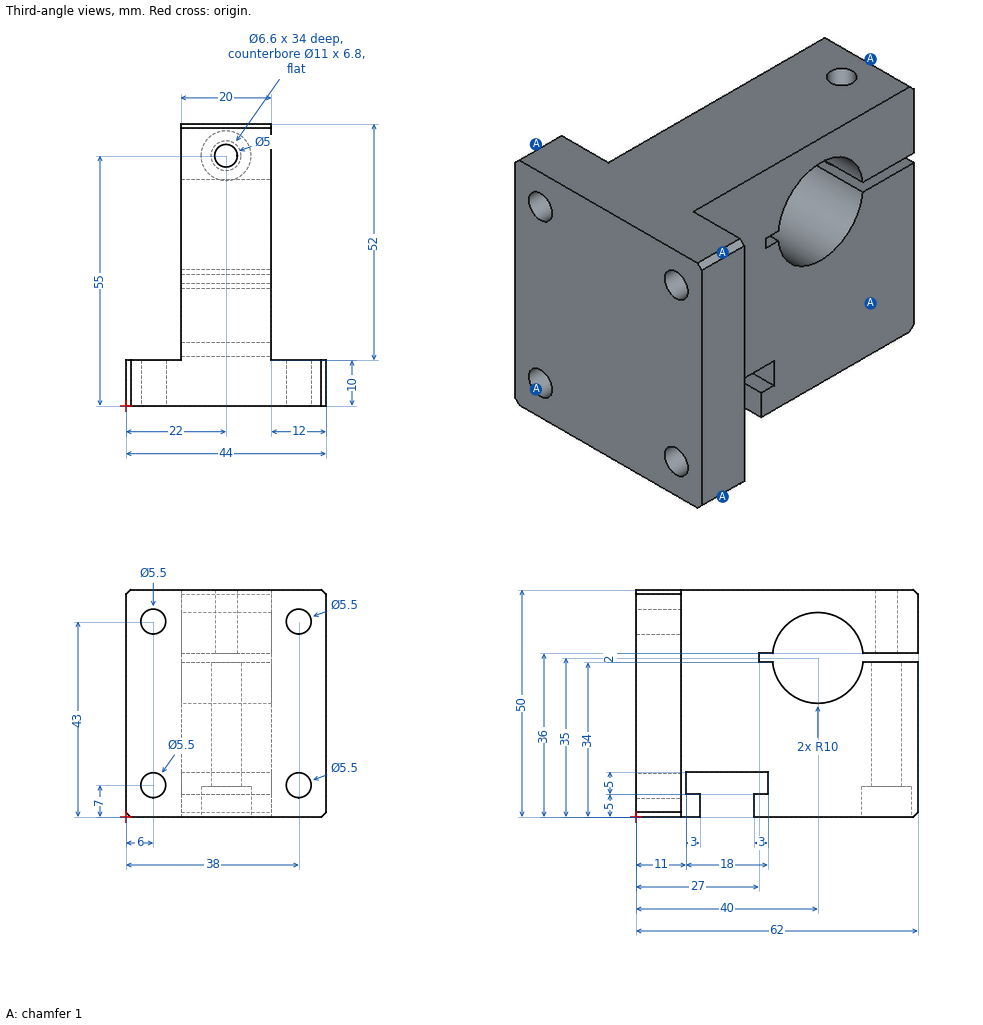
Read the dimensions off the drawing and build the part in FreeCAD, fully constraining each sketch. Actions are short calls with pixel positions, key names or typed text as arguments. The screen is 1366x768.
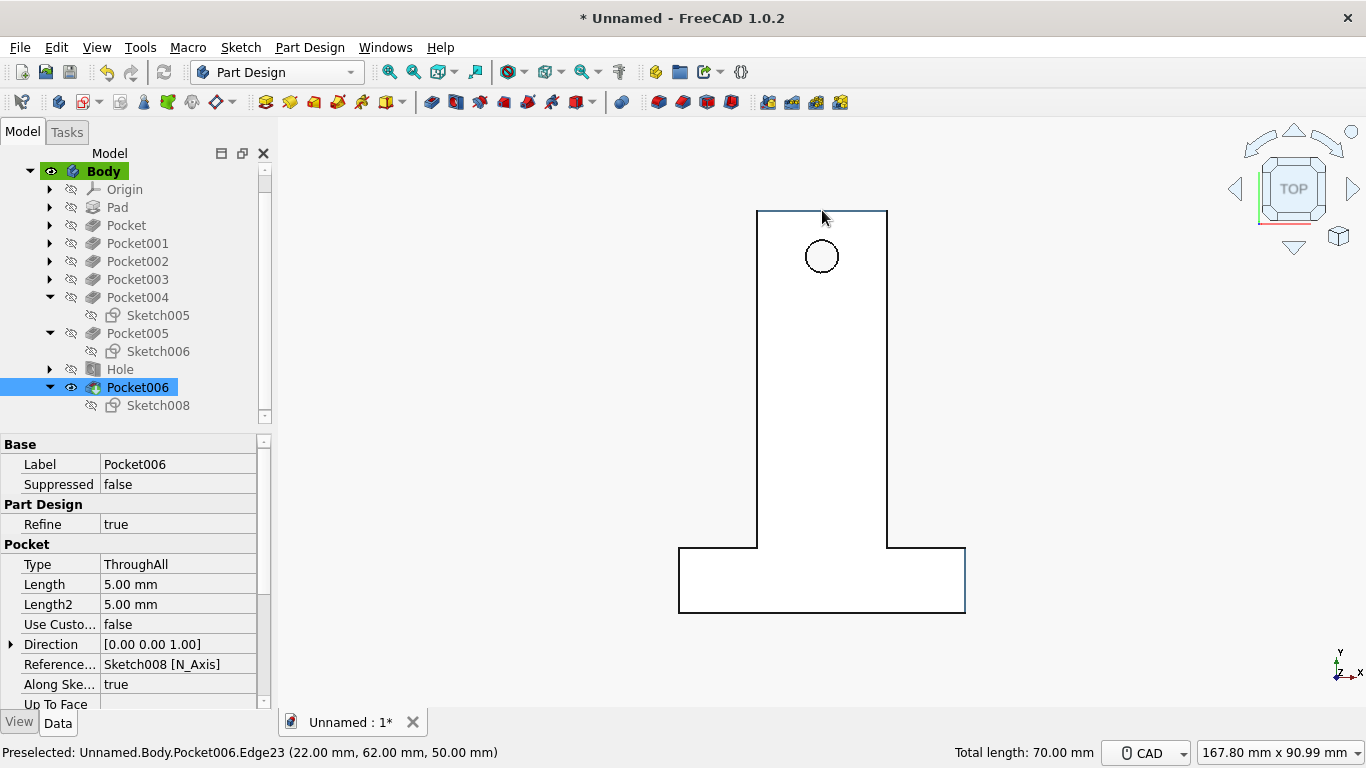
click(679, 580, ctrl)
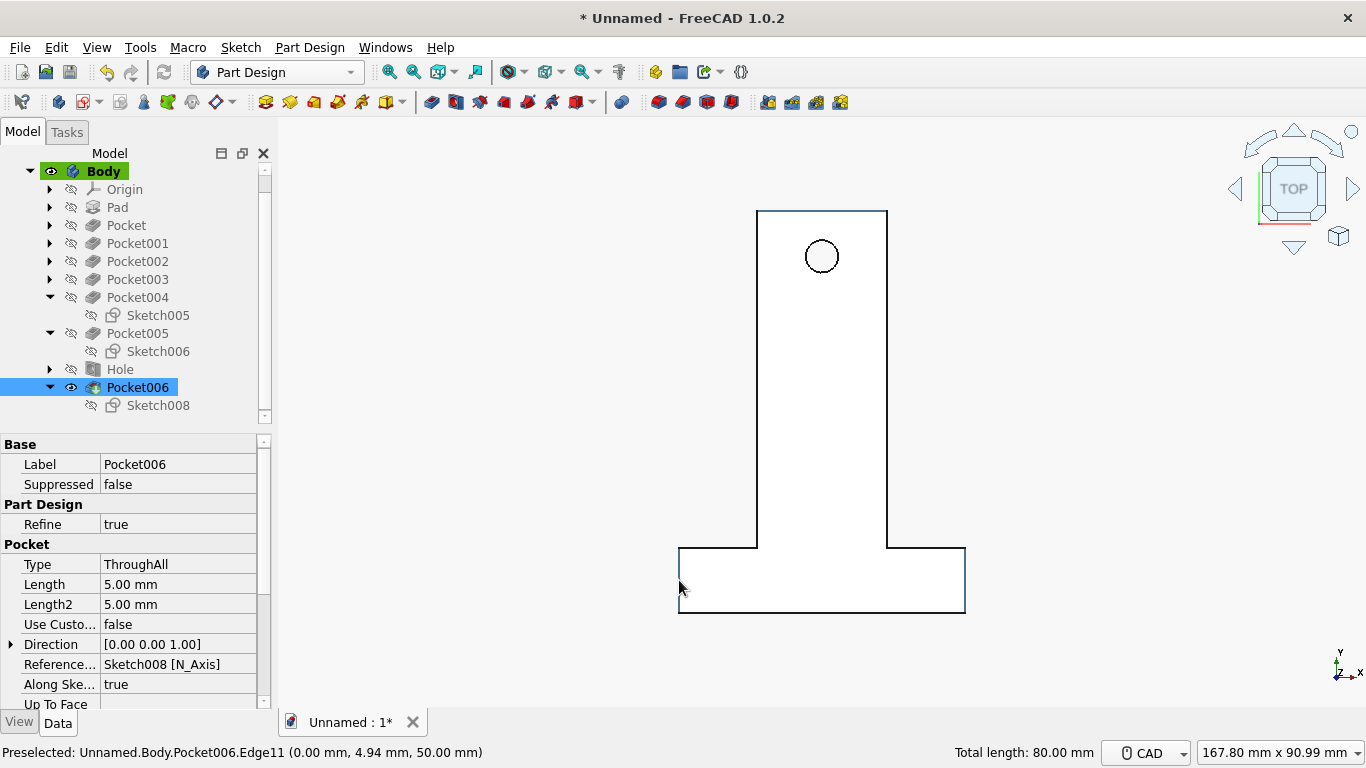
click(684, 102)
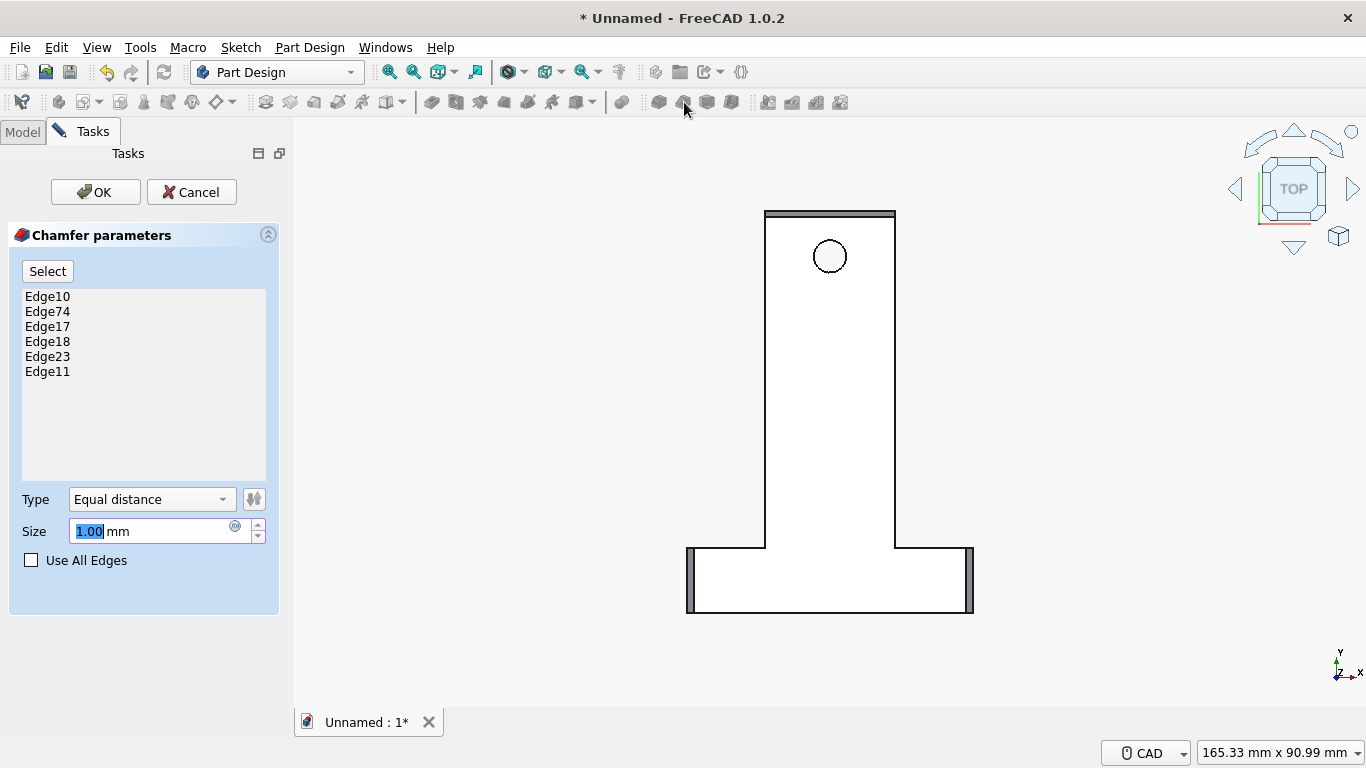
text(1)
key(Tab)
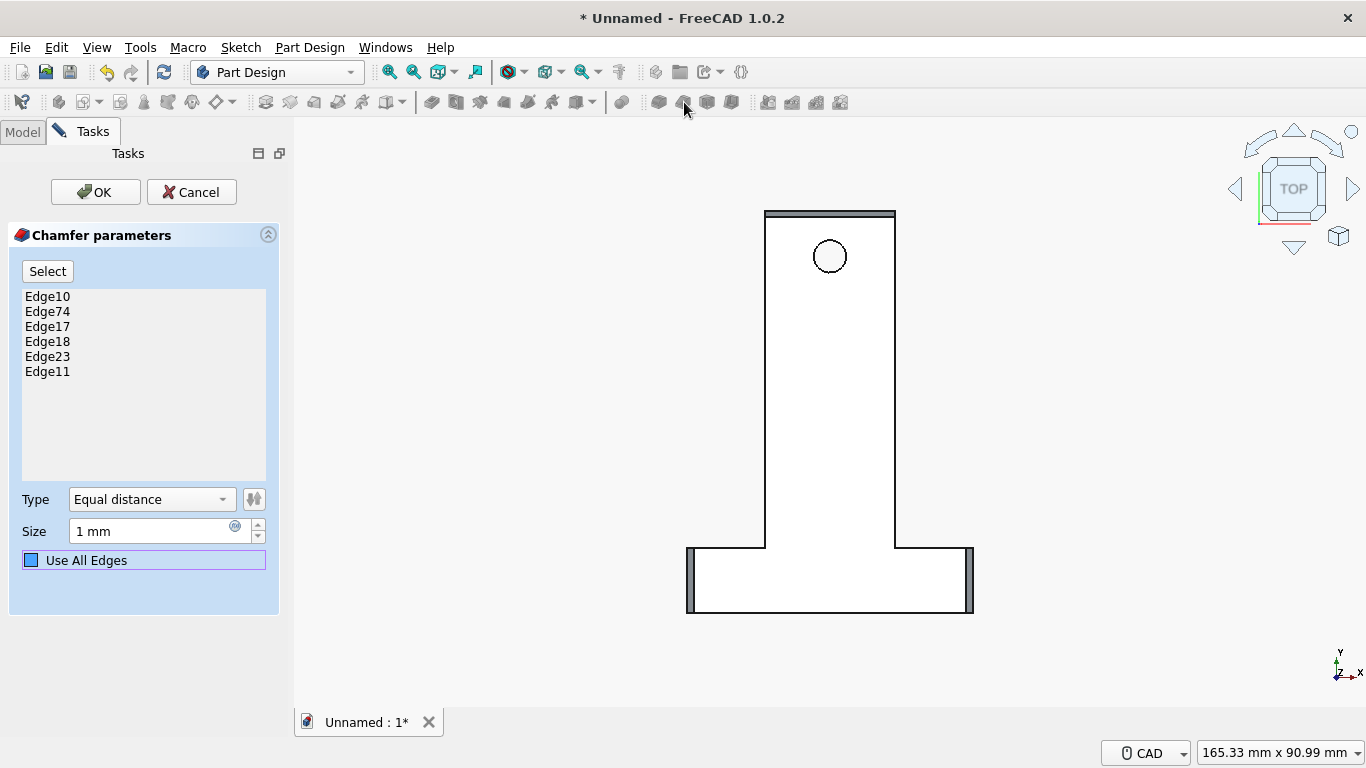
click(96, 192)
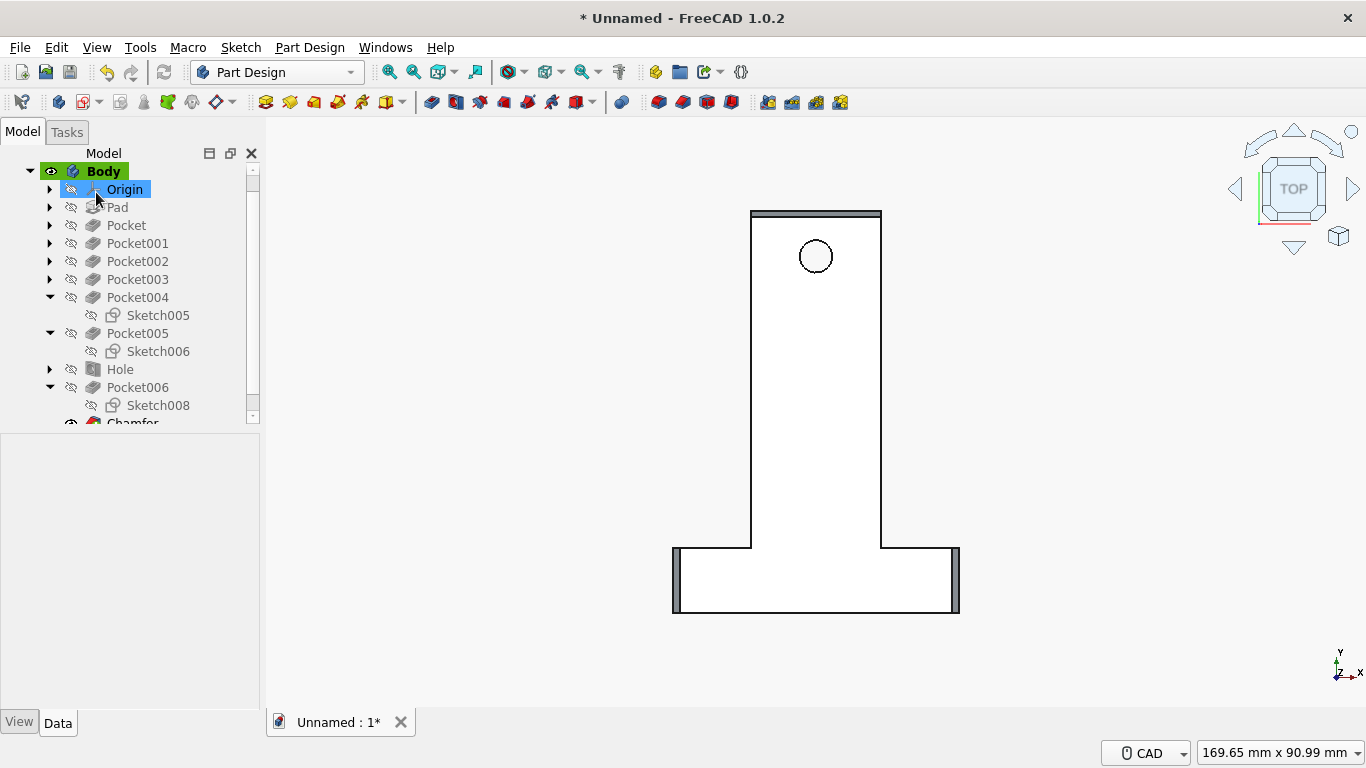
key(0)